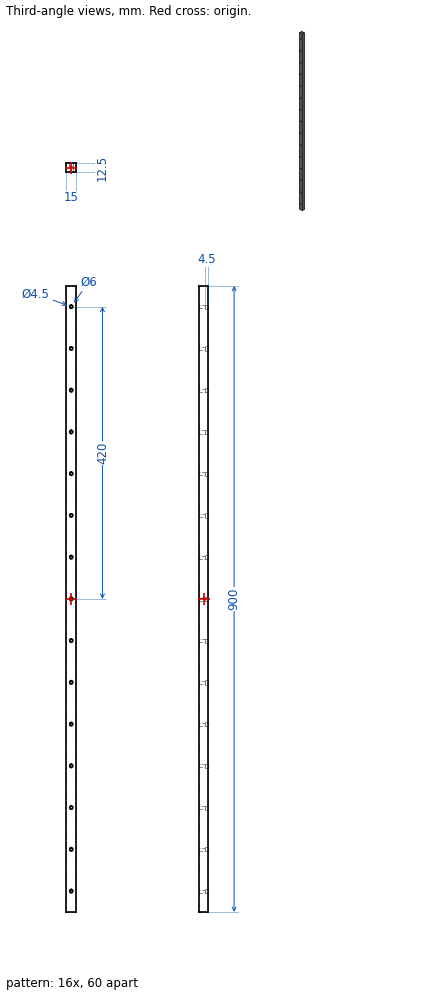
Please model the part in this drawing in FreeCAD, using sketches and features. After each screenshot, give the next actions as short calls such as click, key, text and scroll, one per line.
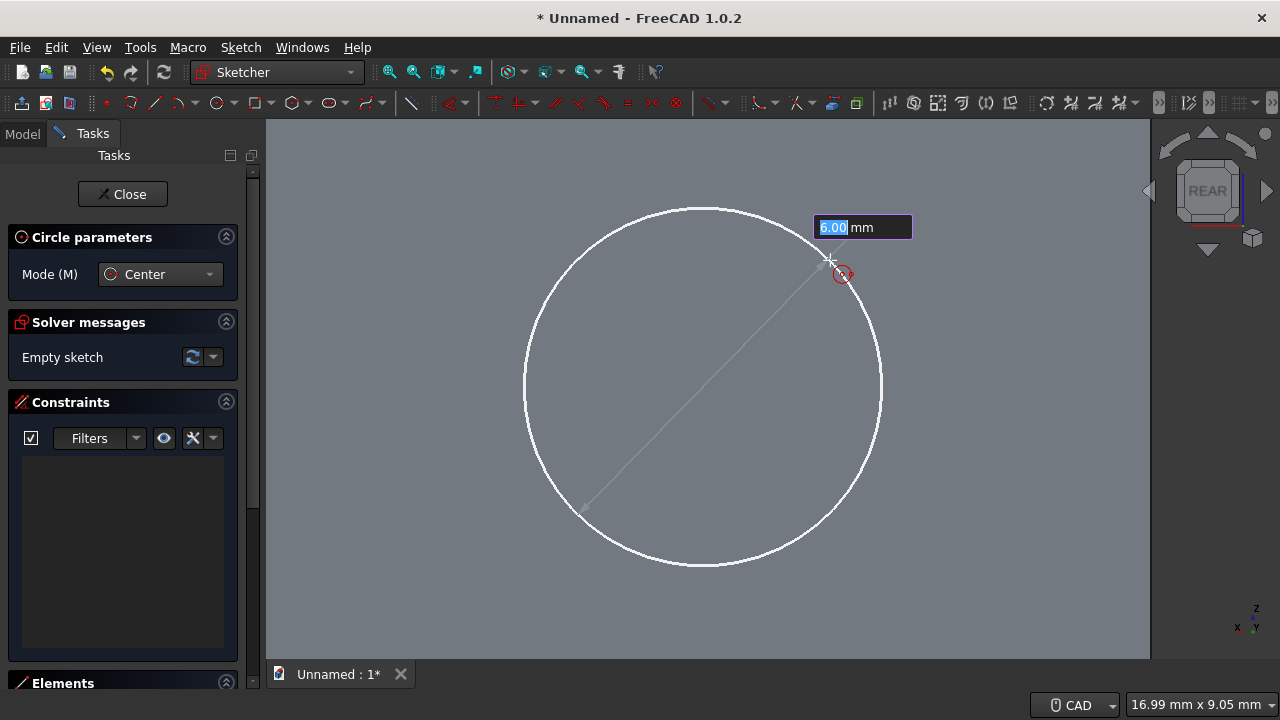
text(6)
key(Return)
key(Escape)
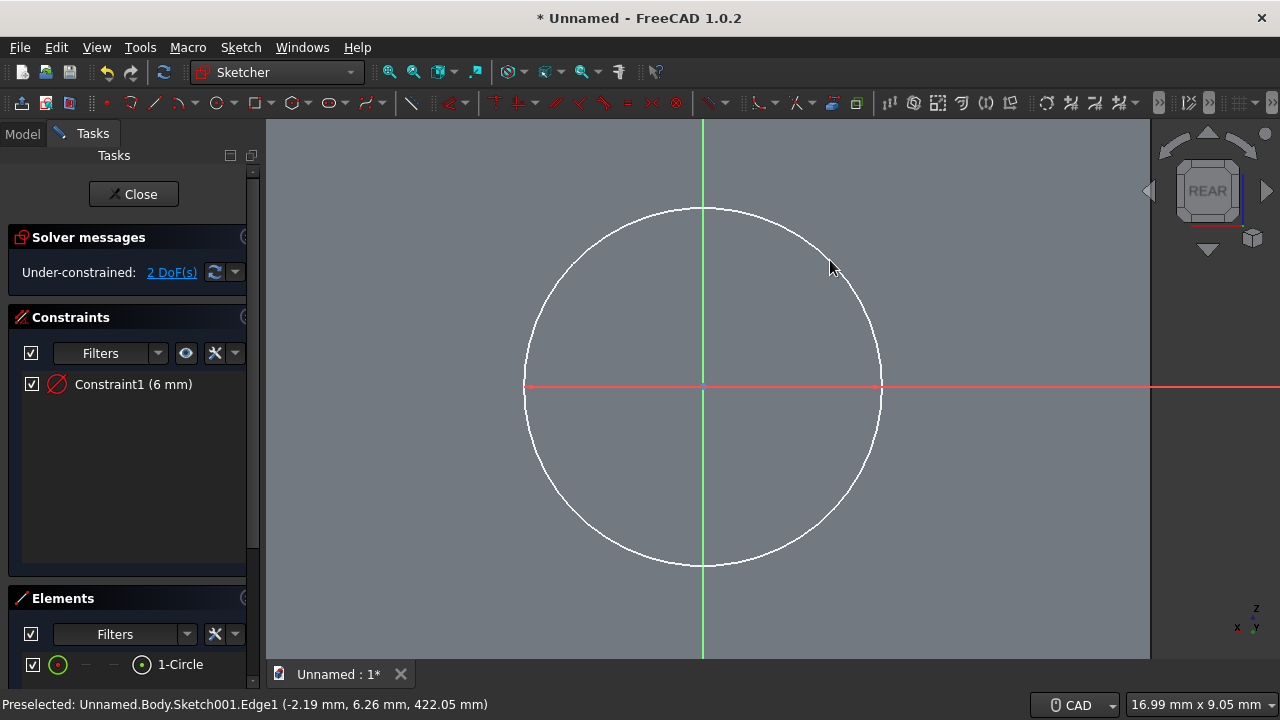
click(703, 387)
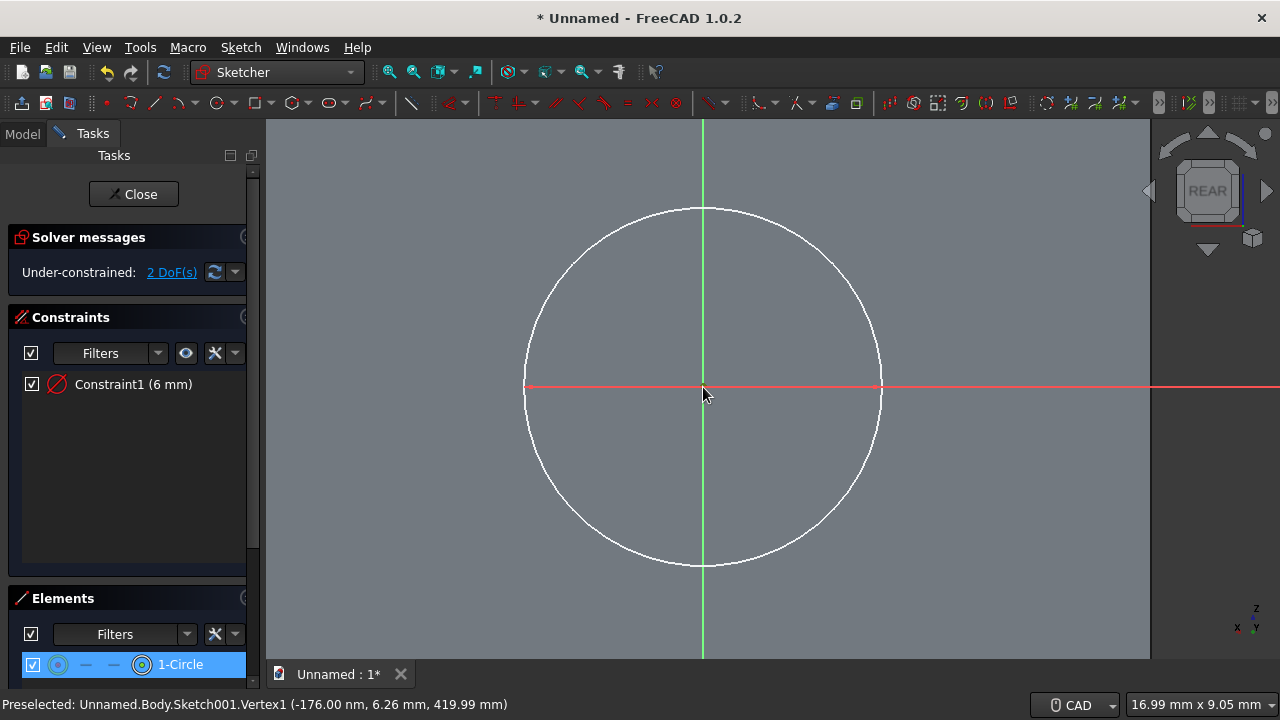
click(703, 596)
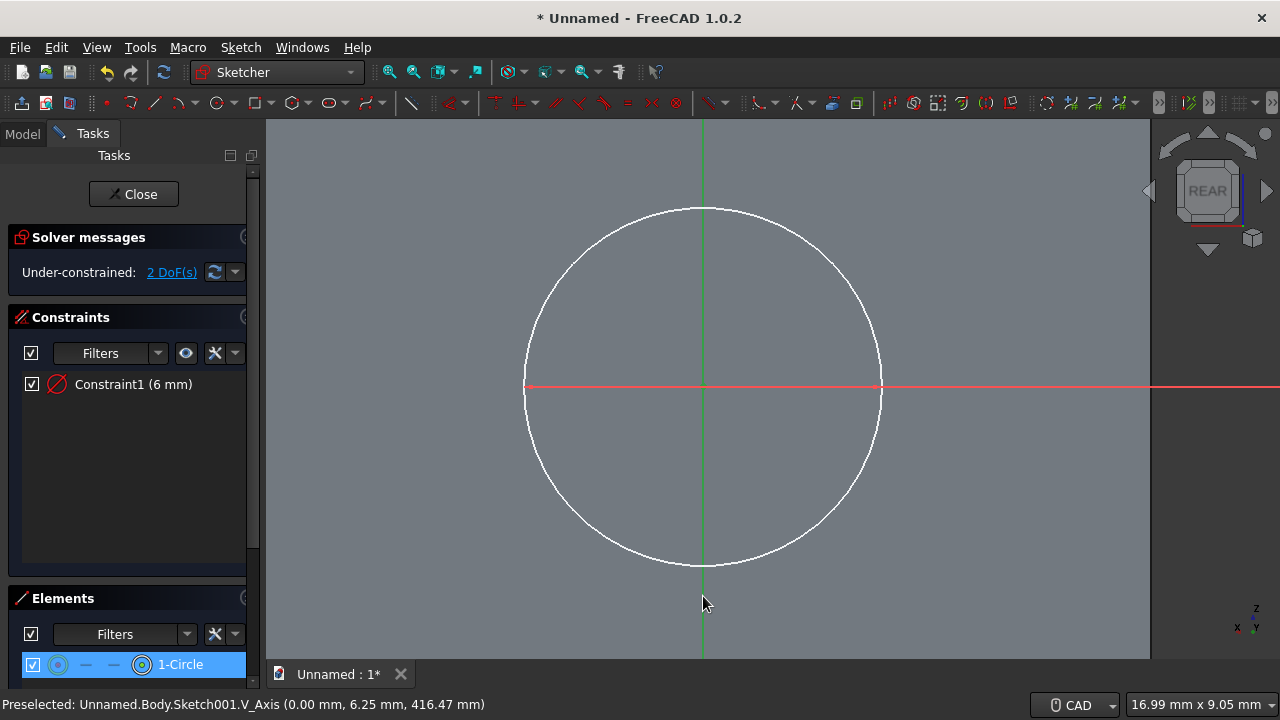
click(496, 104)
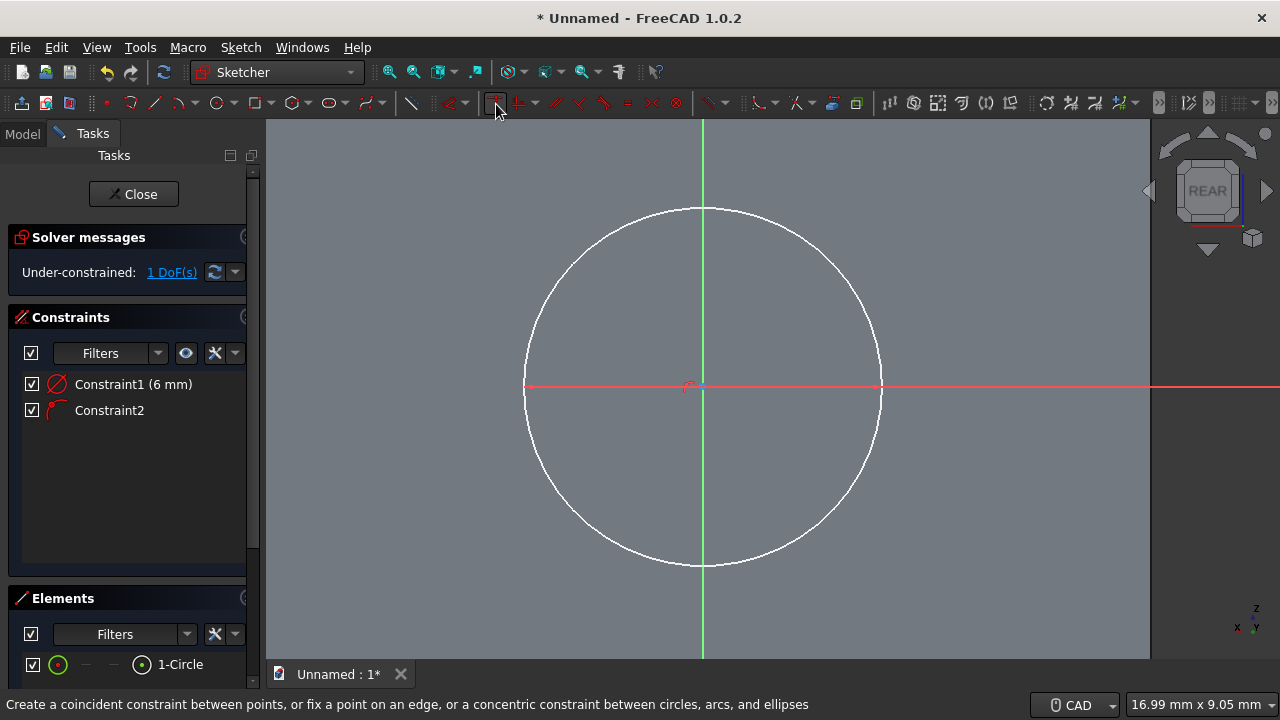
click(703, 387)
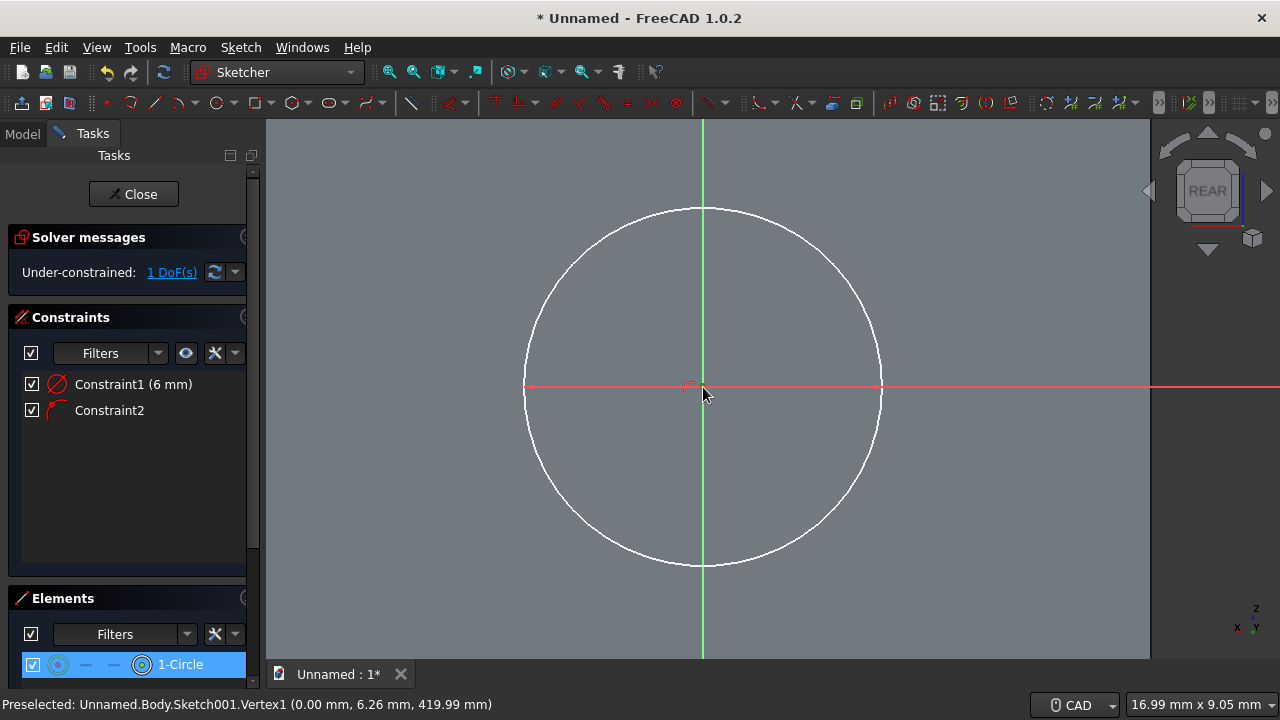
click(468, 104)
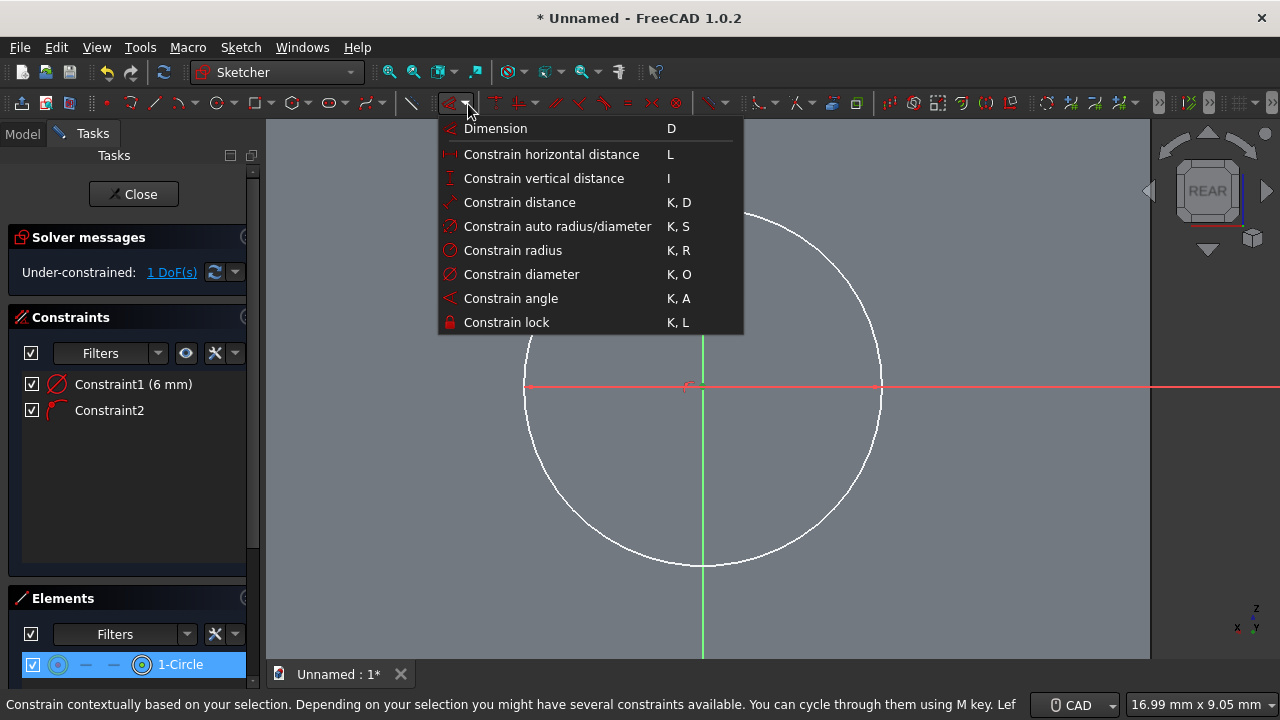
click(591, 178)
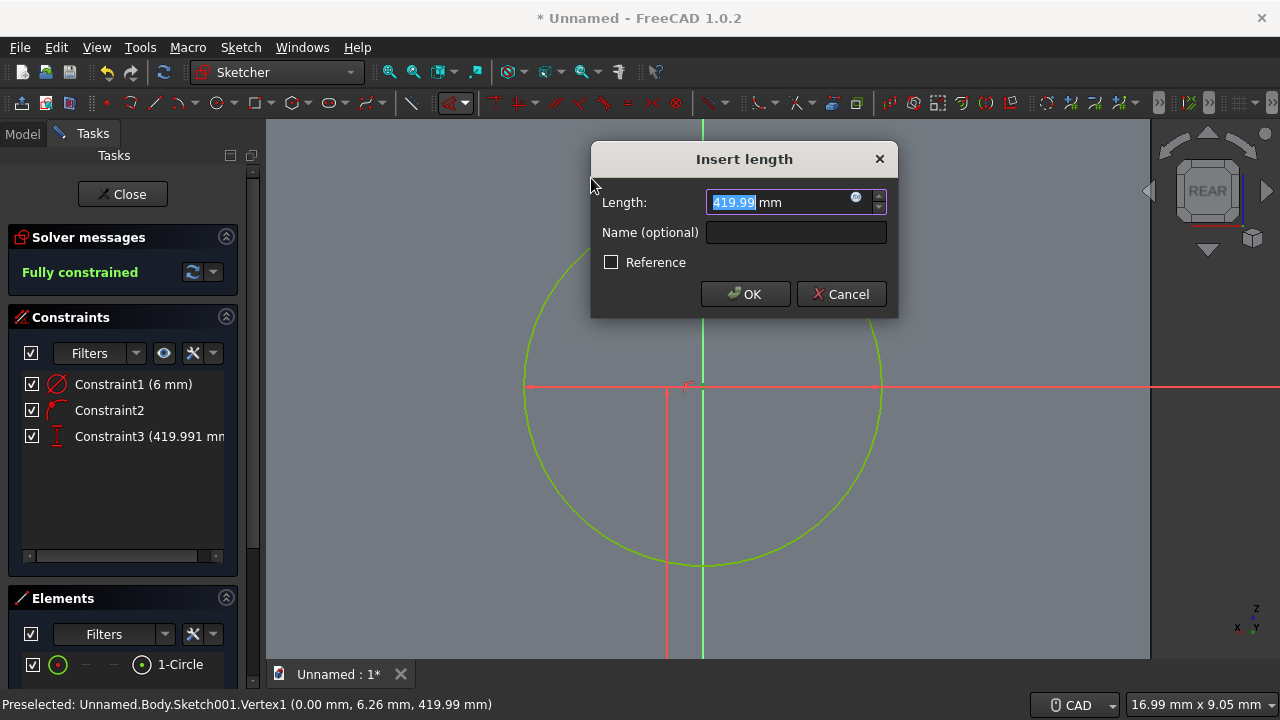
text(420)
key(Return)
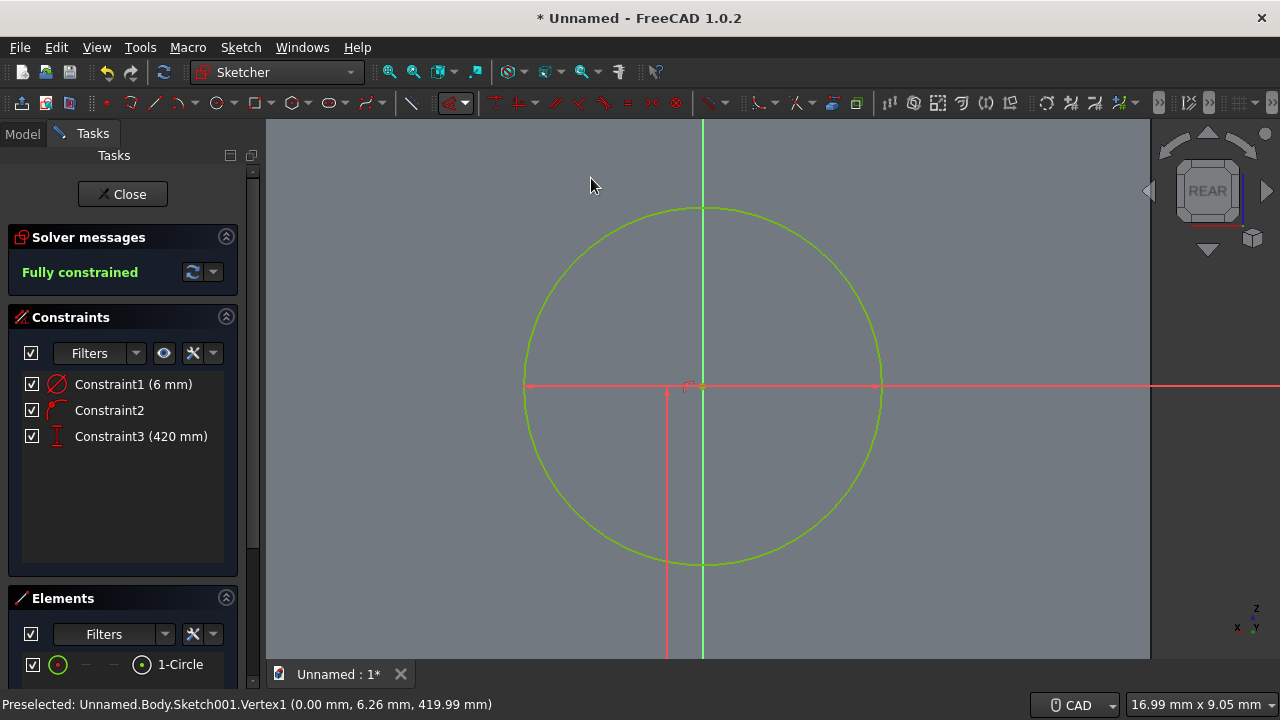
click(123, 194)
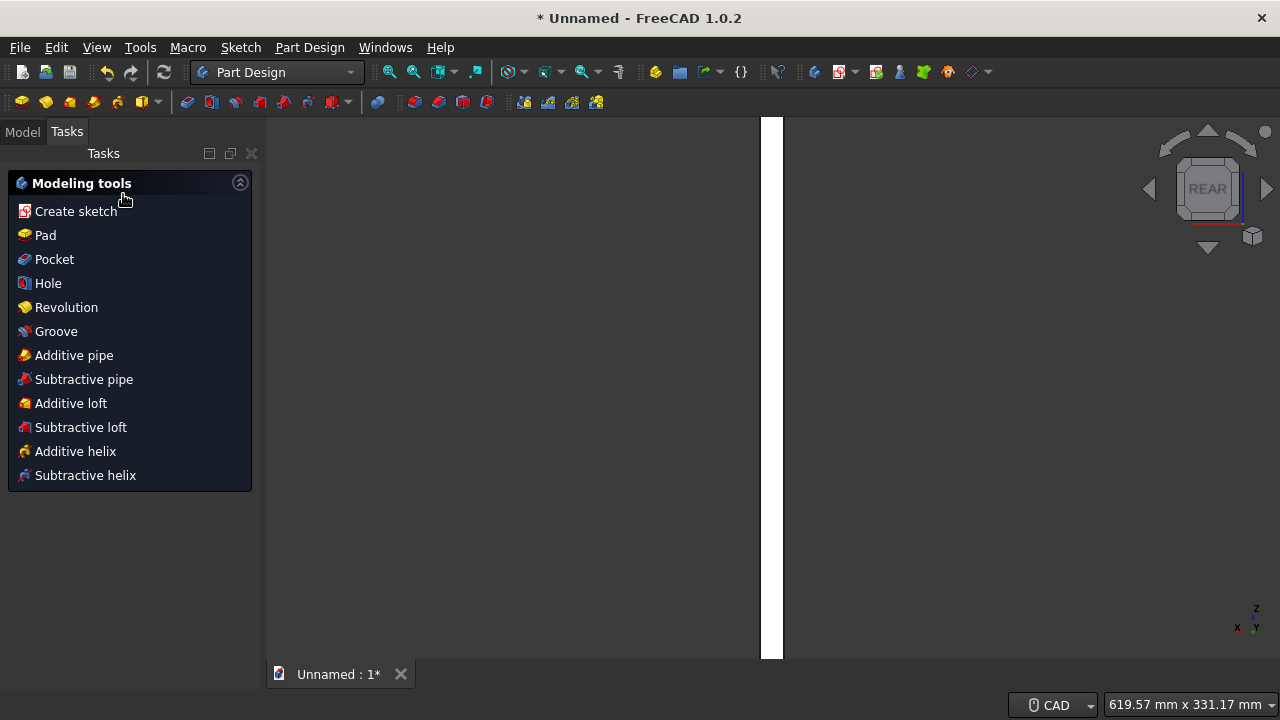
click(188, 102)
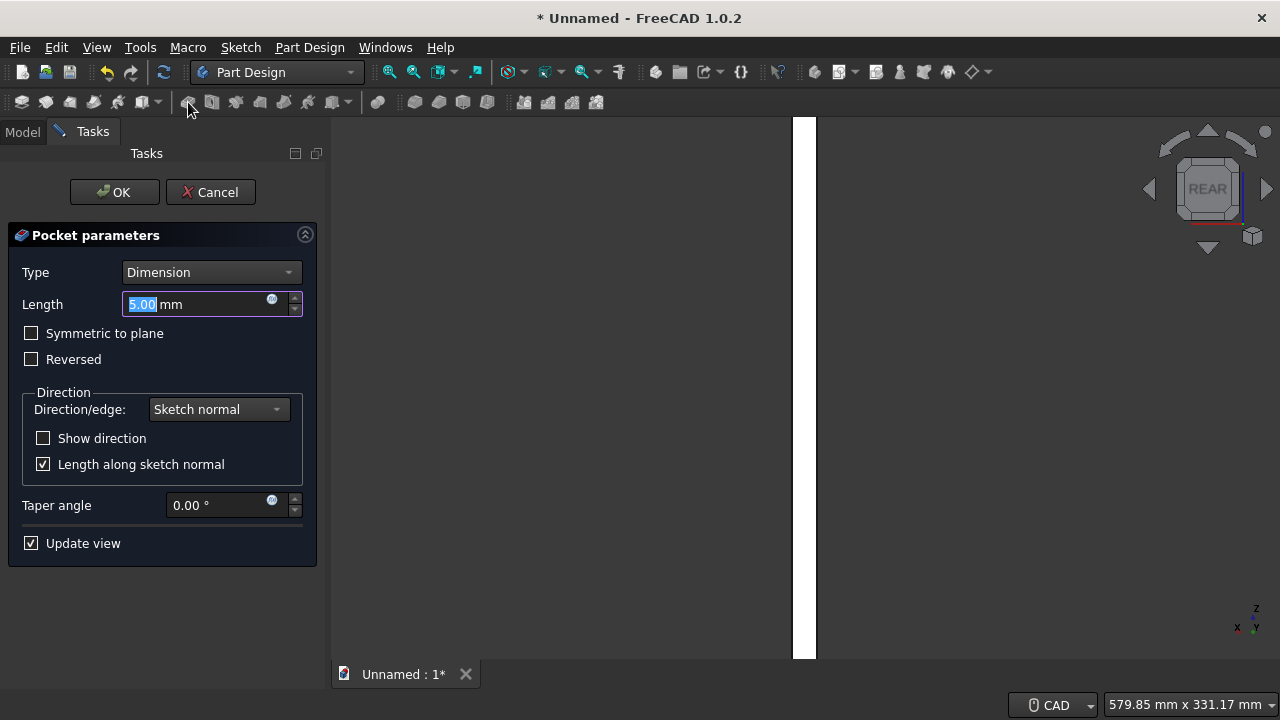
text(4.5)
key(Tab)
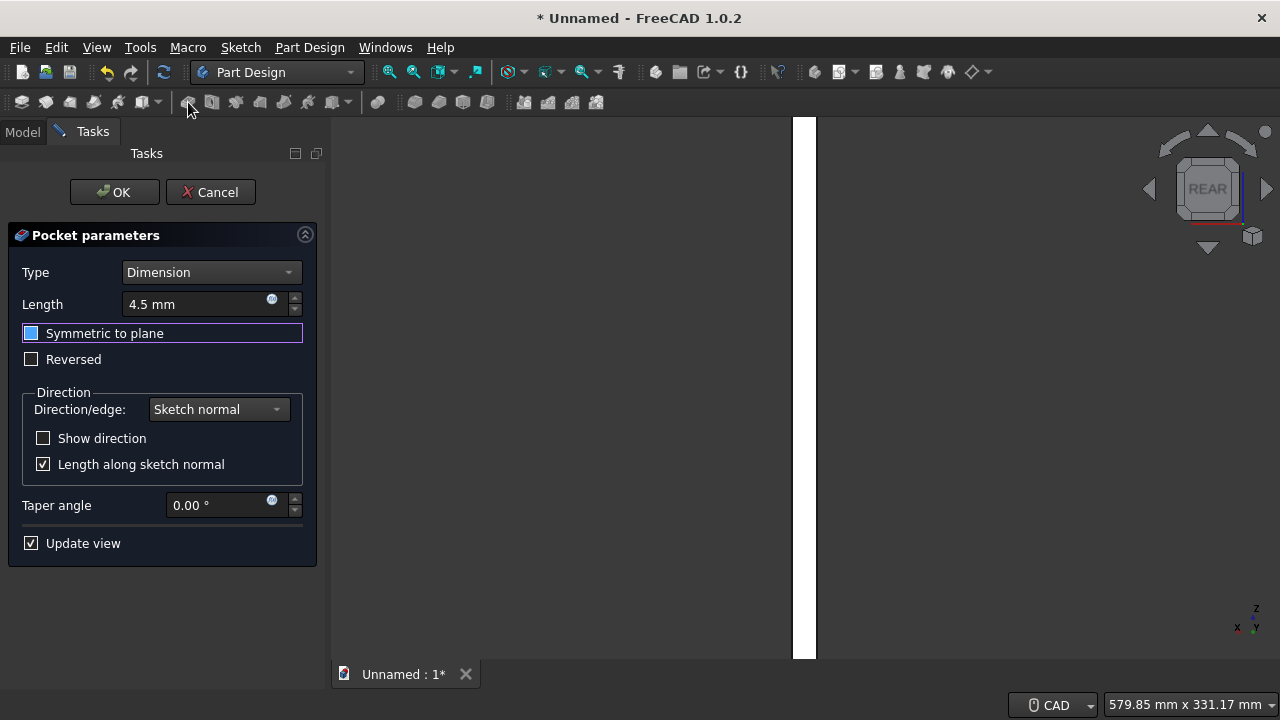
click(115, 192)